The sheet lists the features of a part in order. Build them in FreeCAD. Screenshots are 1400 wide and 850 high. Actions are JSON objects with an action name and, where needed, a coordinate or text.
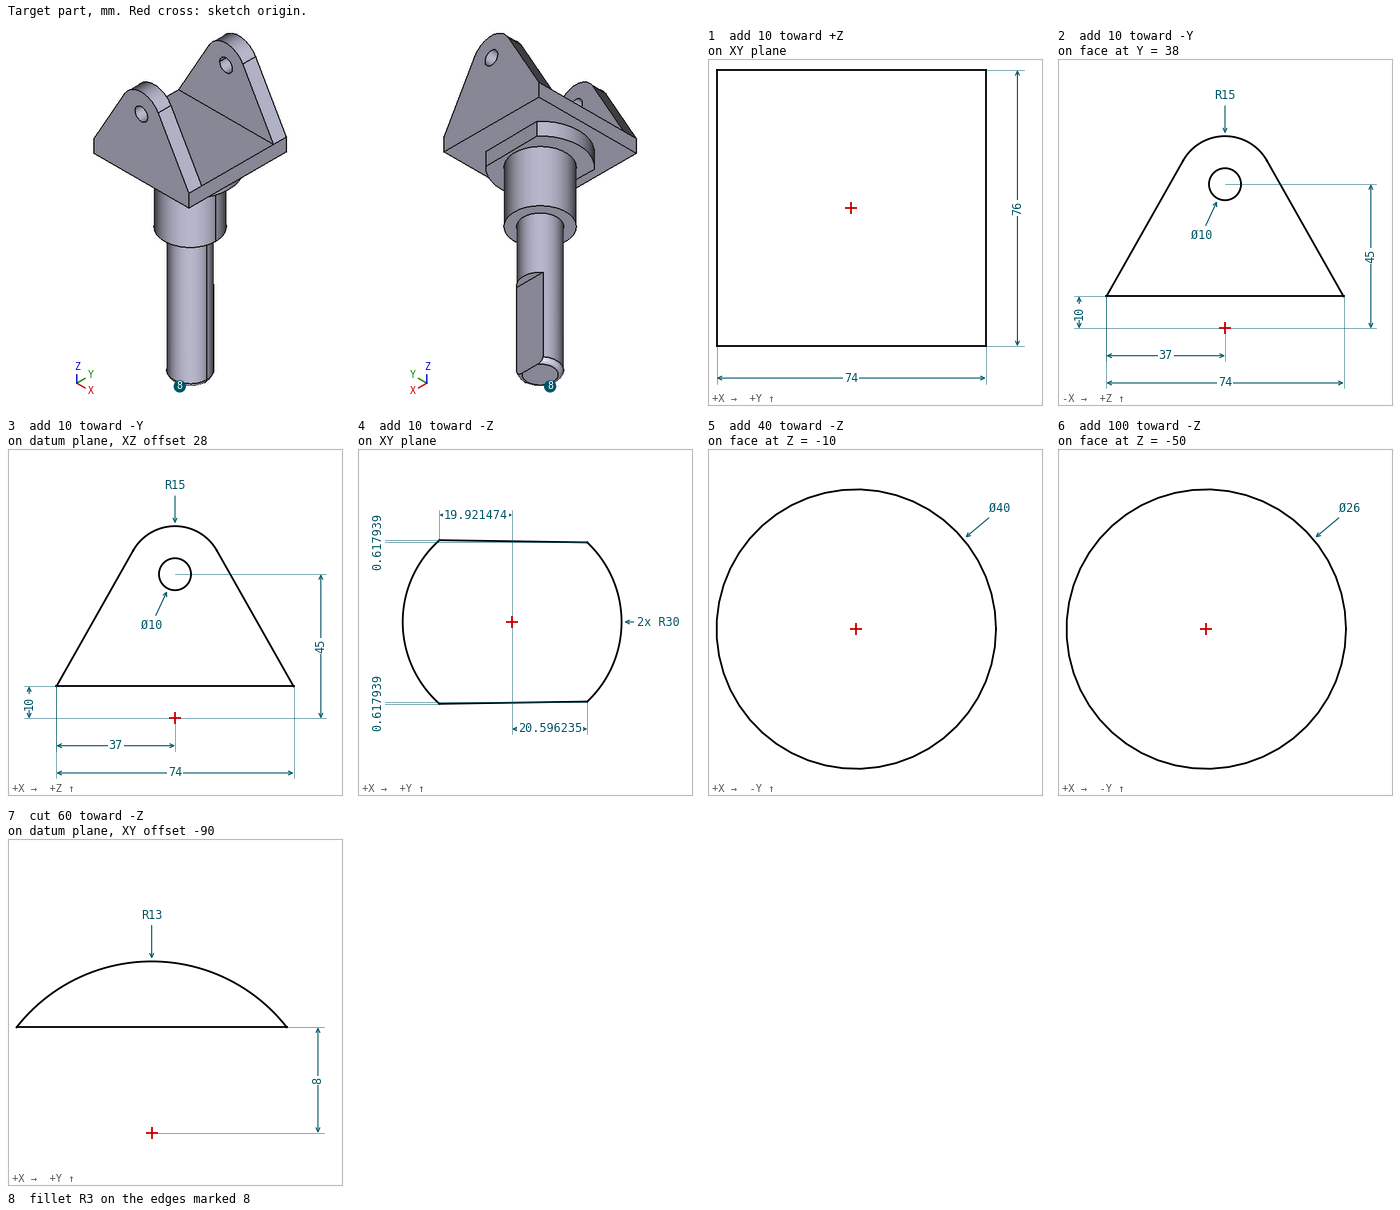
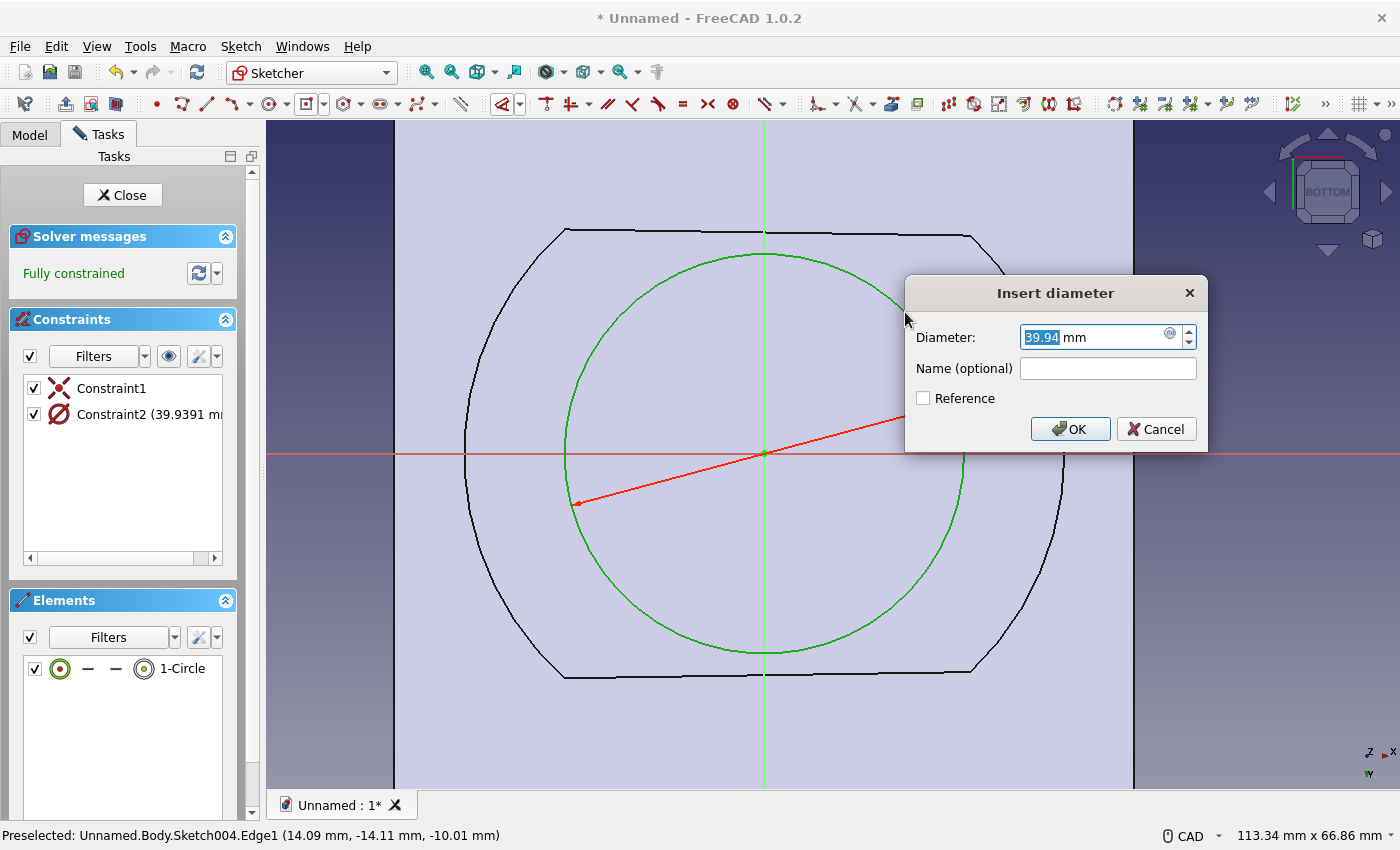
{"action": "type", "text": "40"}
{"action": "key", "text": "Return"}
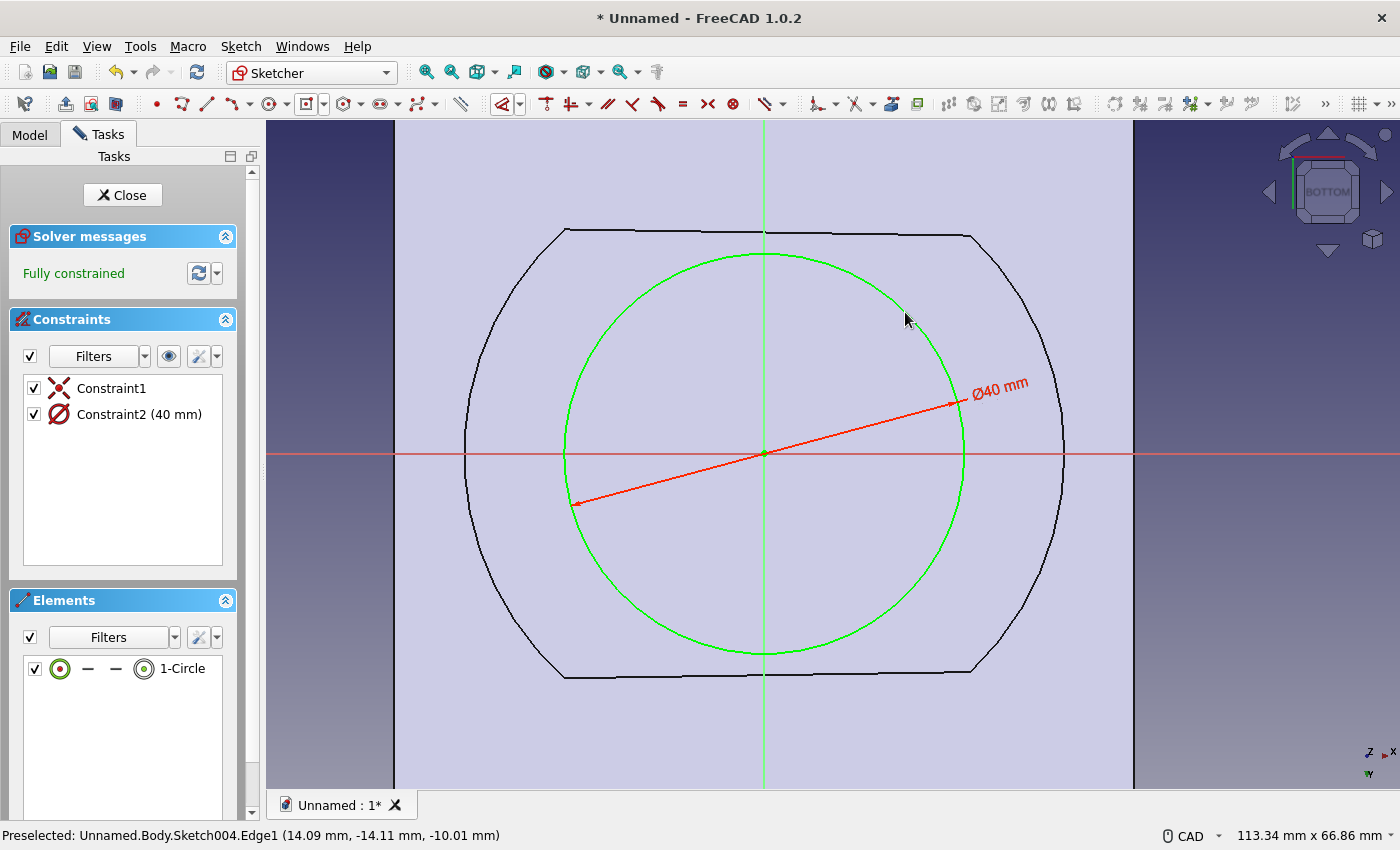
{"action": "left_click", "coordinate": [123, 195]}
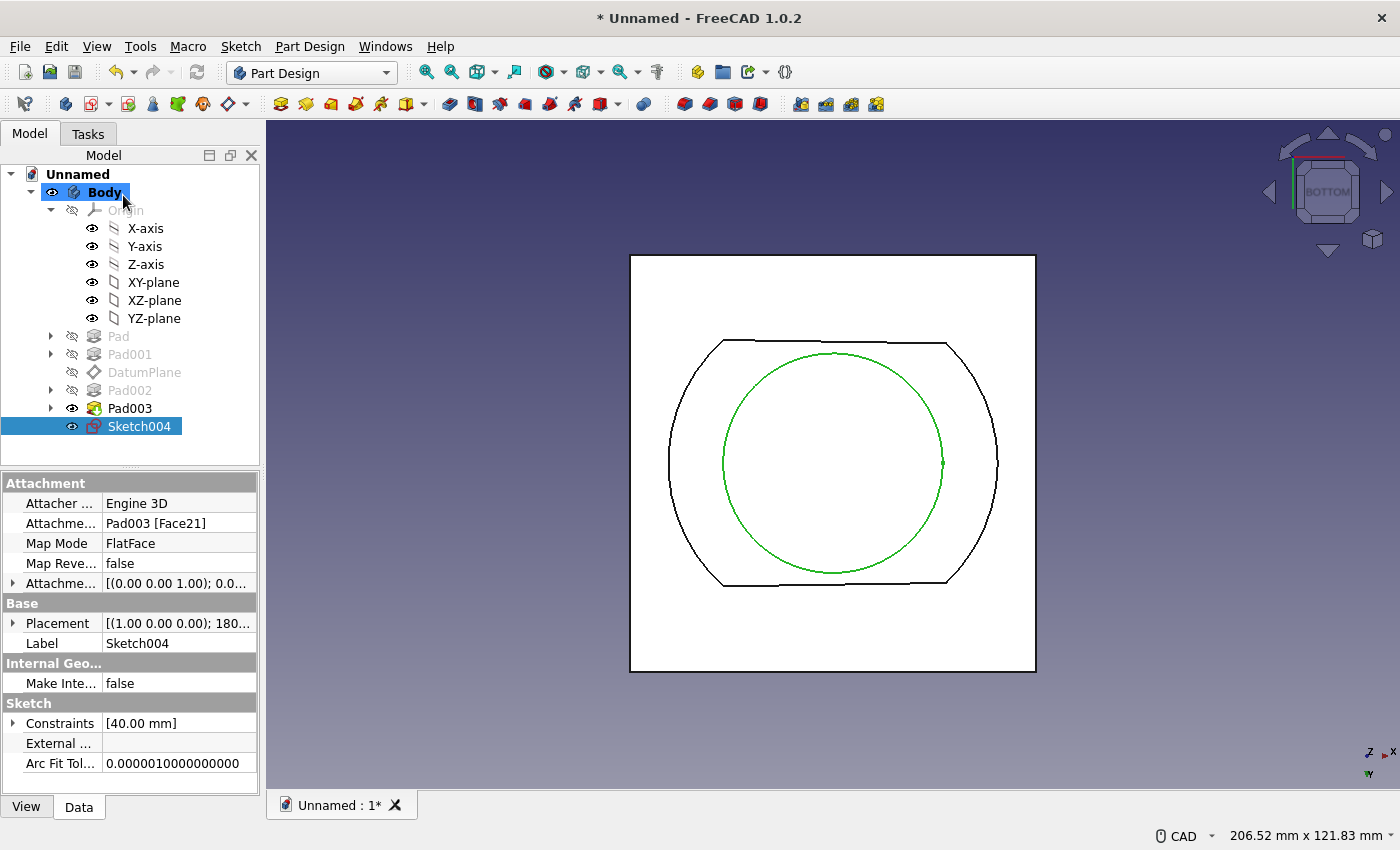
{"action": "left_click", "coordinate": [281, 104]}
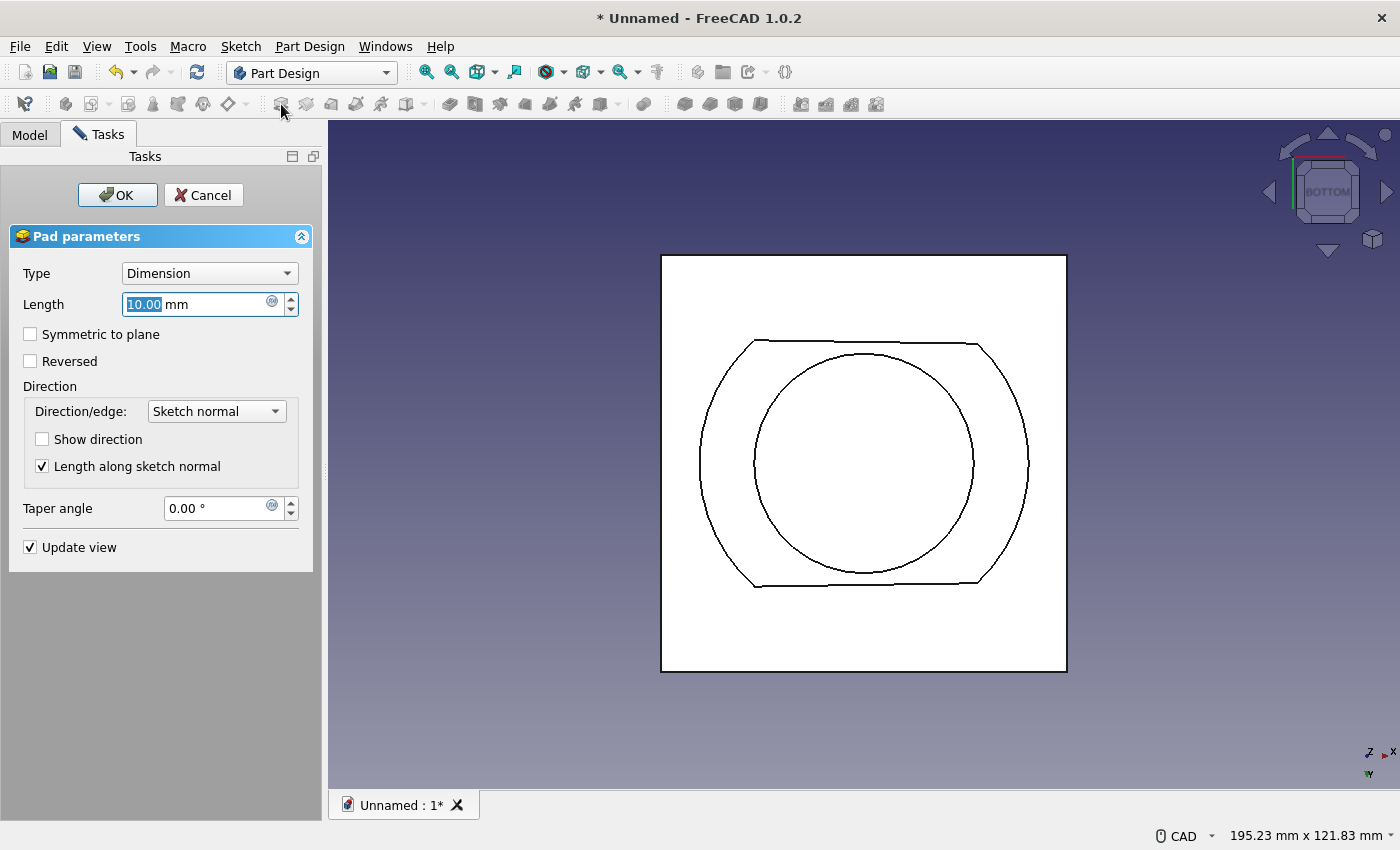
{"action": "type", "text": "40"}
{"action": "key", "text": "Tab"}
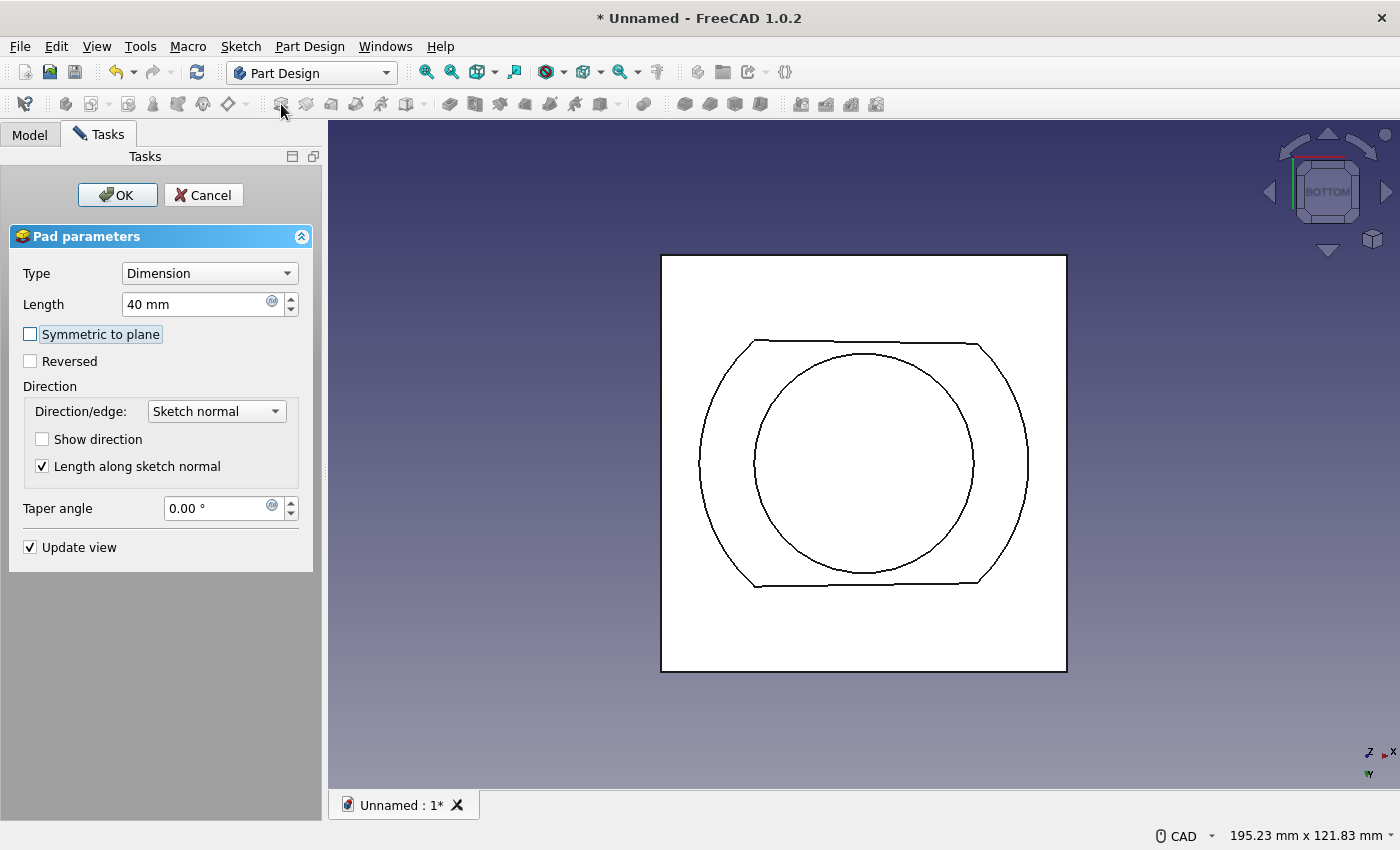
{"action": "left_click", "coordinate": [118, 195]}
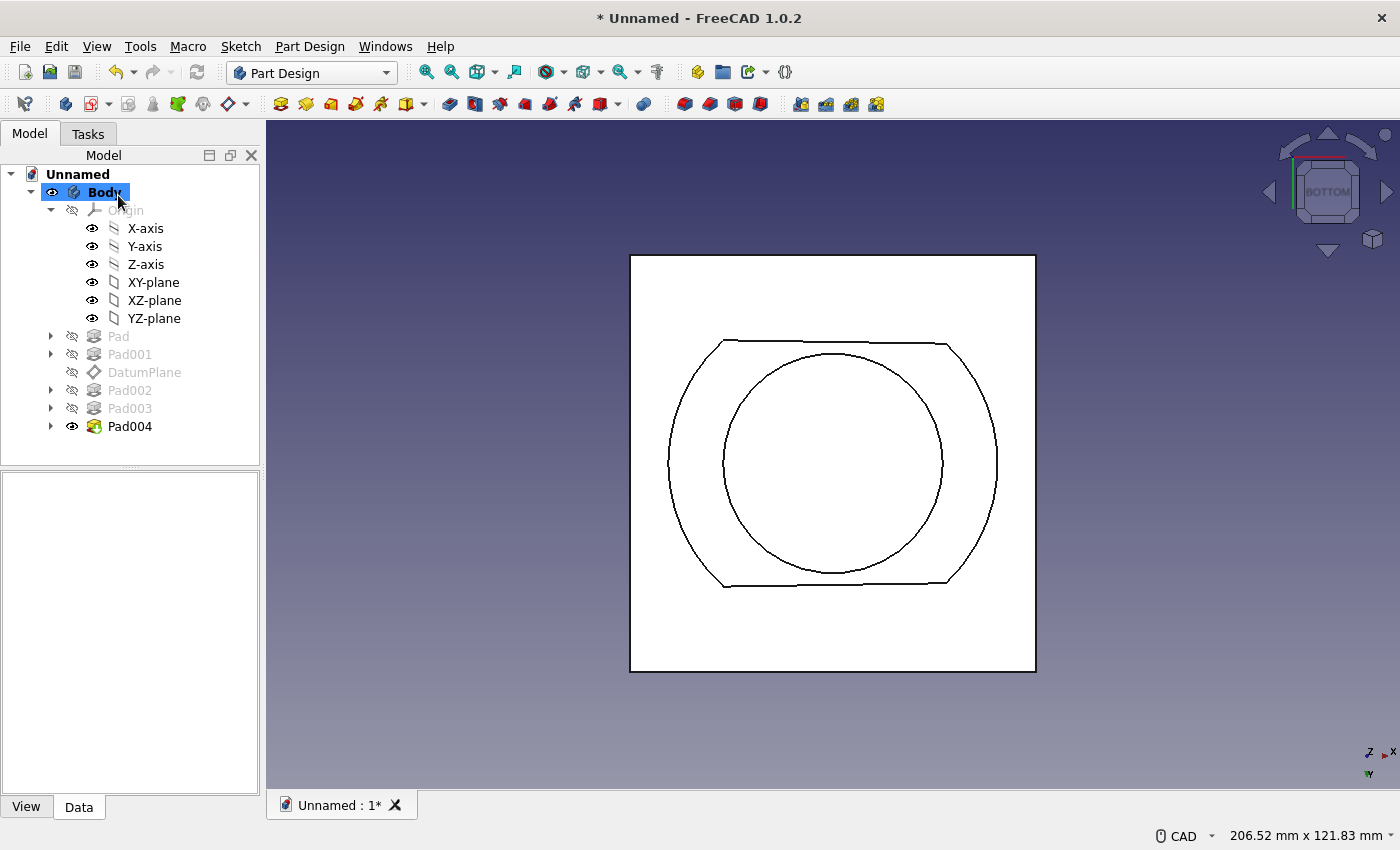
{"action": "left_click", "coordinate": [833, 462]}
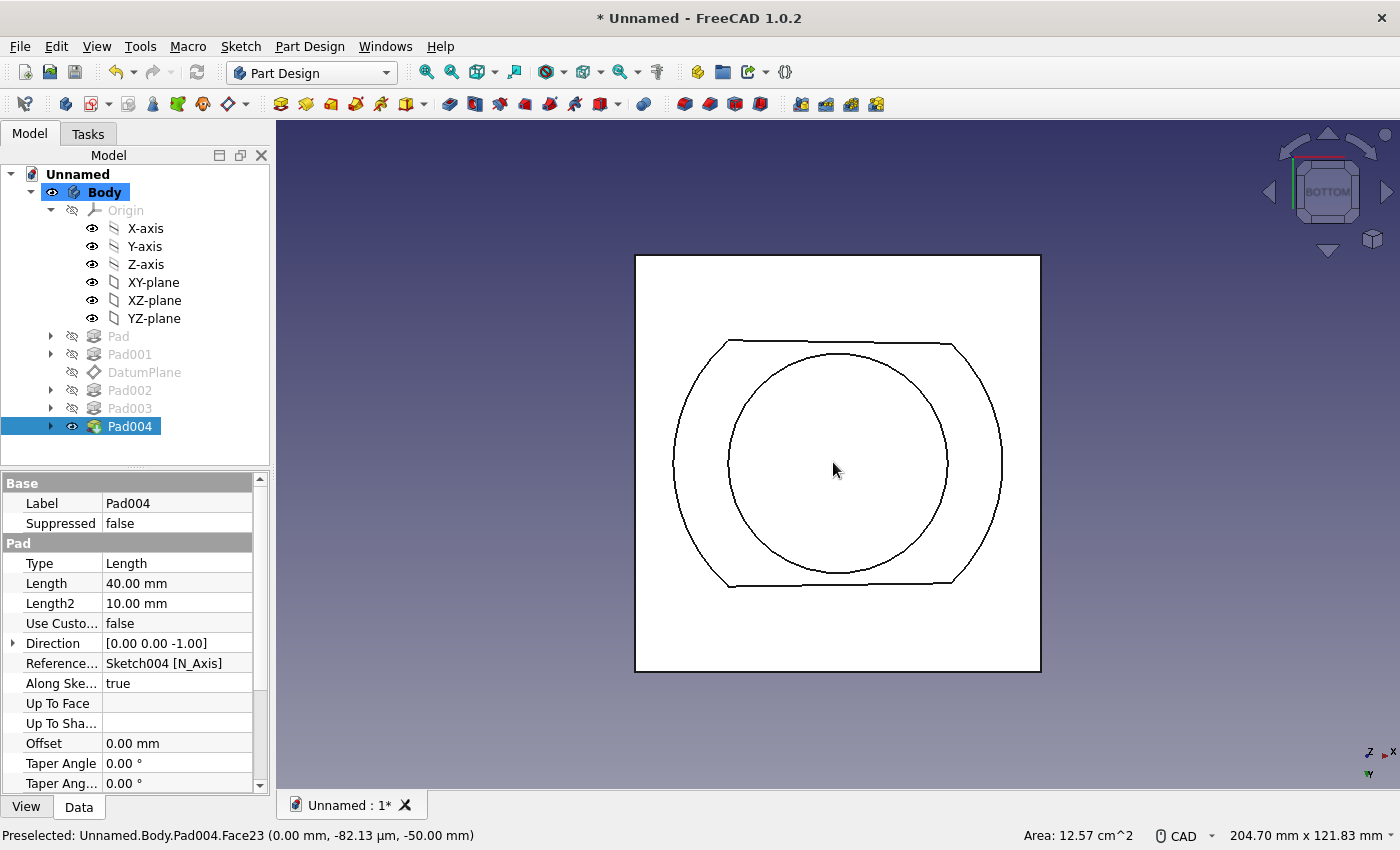
{"action": "left_click", "coordinate": [90, 104]}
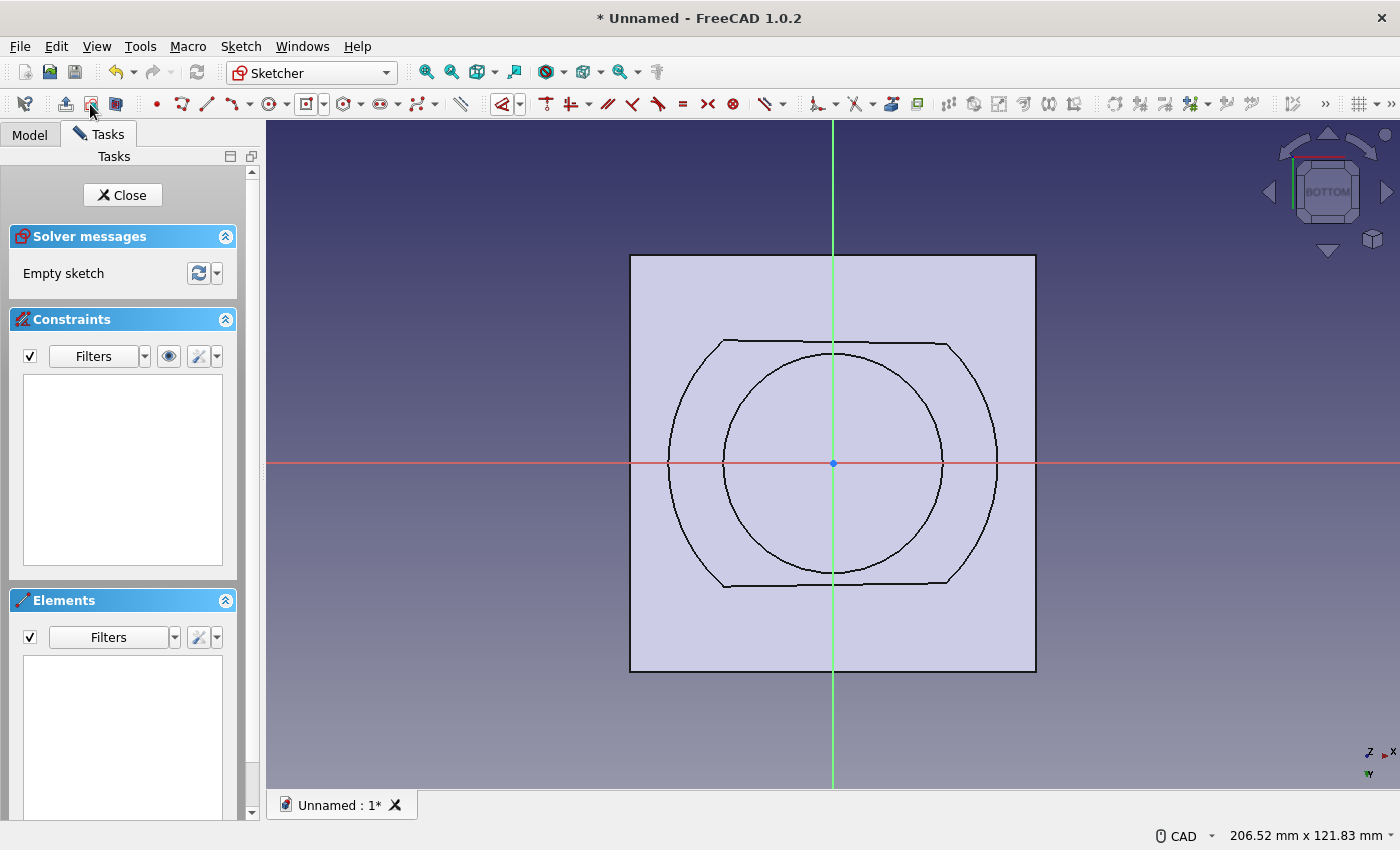
{"action": "scroll", "coordinate": [863, 467], "scroll_direction": "up", "scroll_amount": 6}